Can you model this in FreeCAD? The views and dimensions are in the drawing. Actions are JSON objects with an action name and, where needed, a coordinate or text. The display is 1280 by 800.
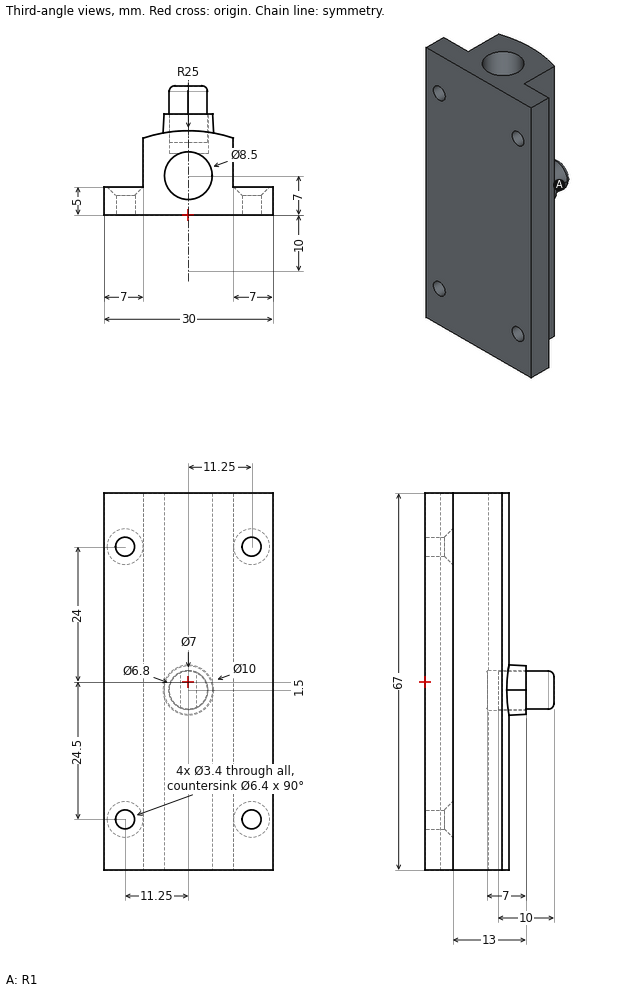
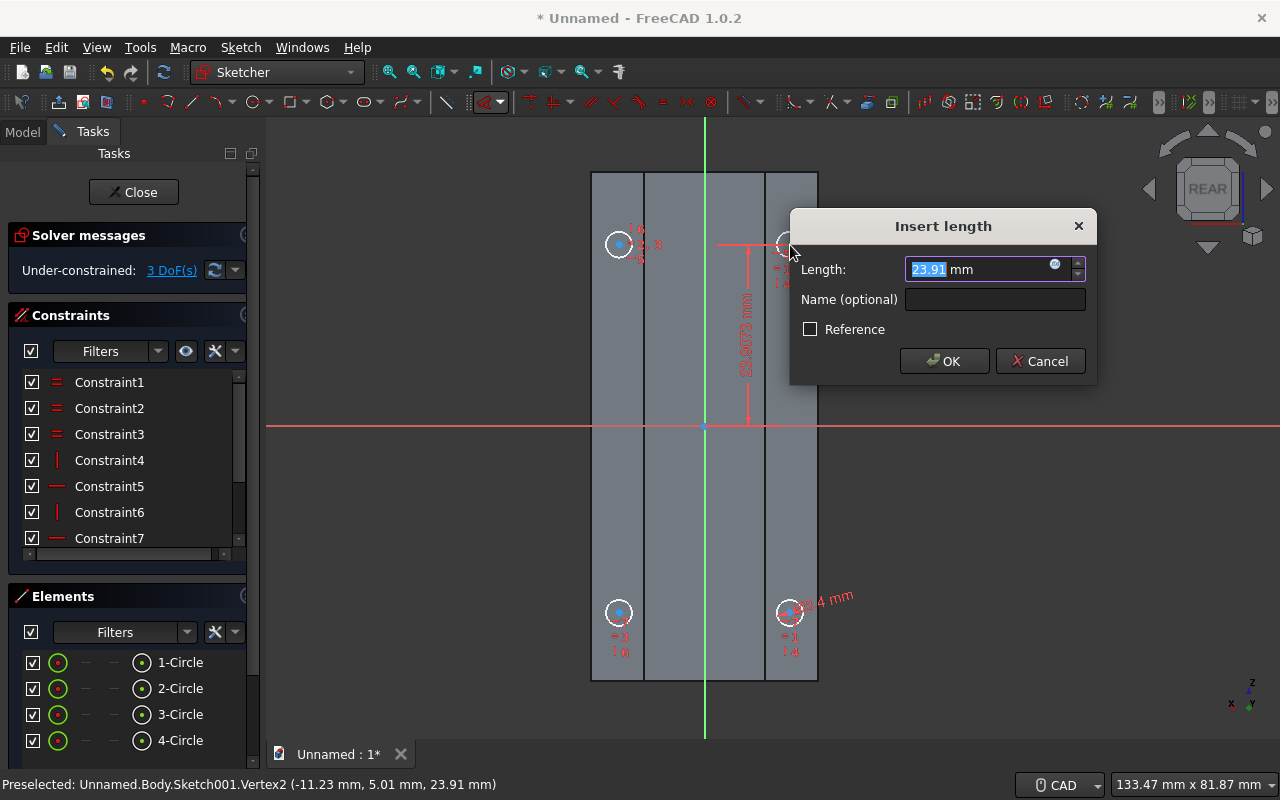
{"action": "type", "text": "24"}
{"action": "key", "text": "Return"}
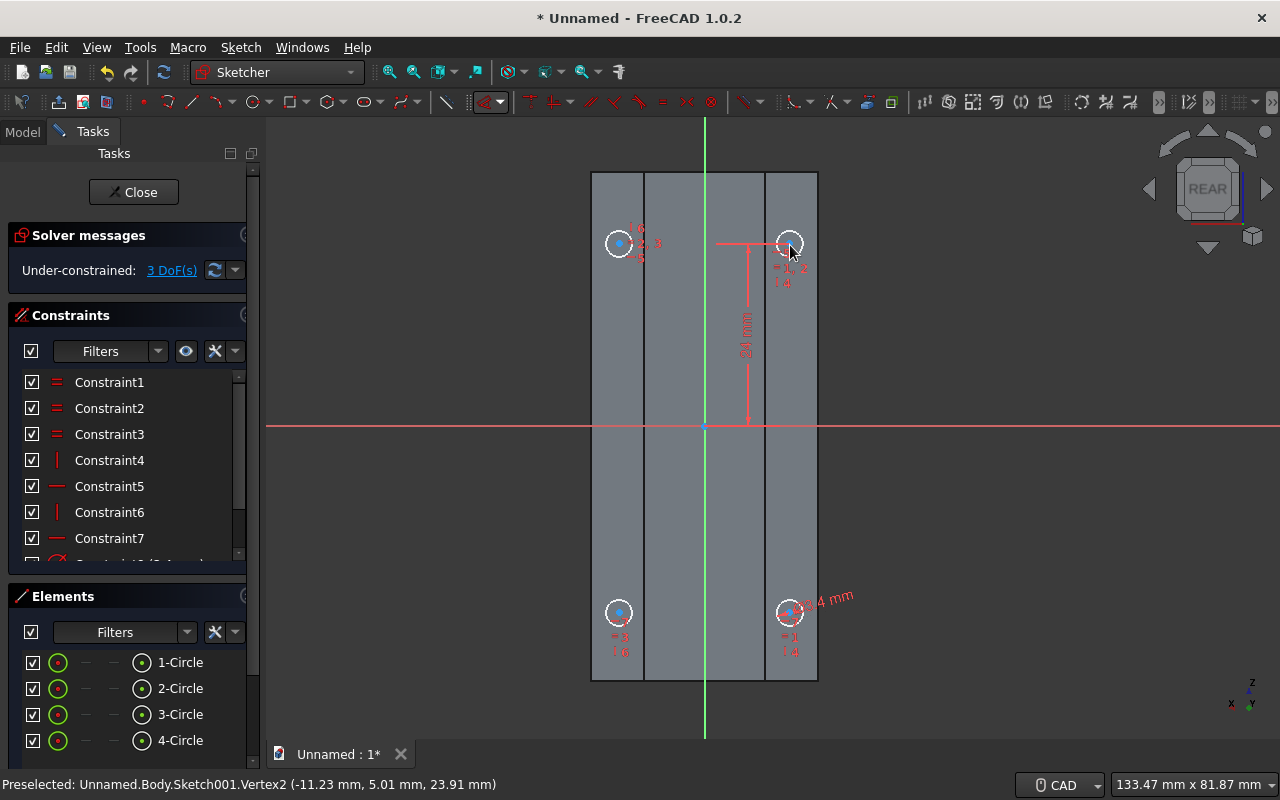
{"action": "left_click", "coordinate": [790, 613]}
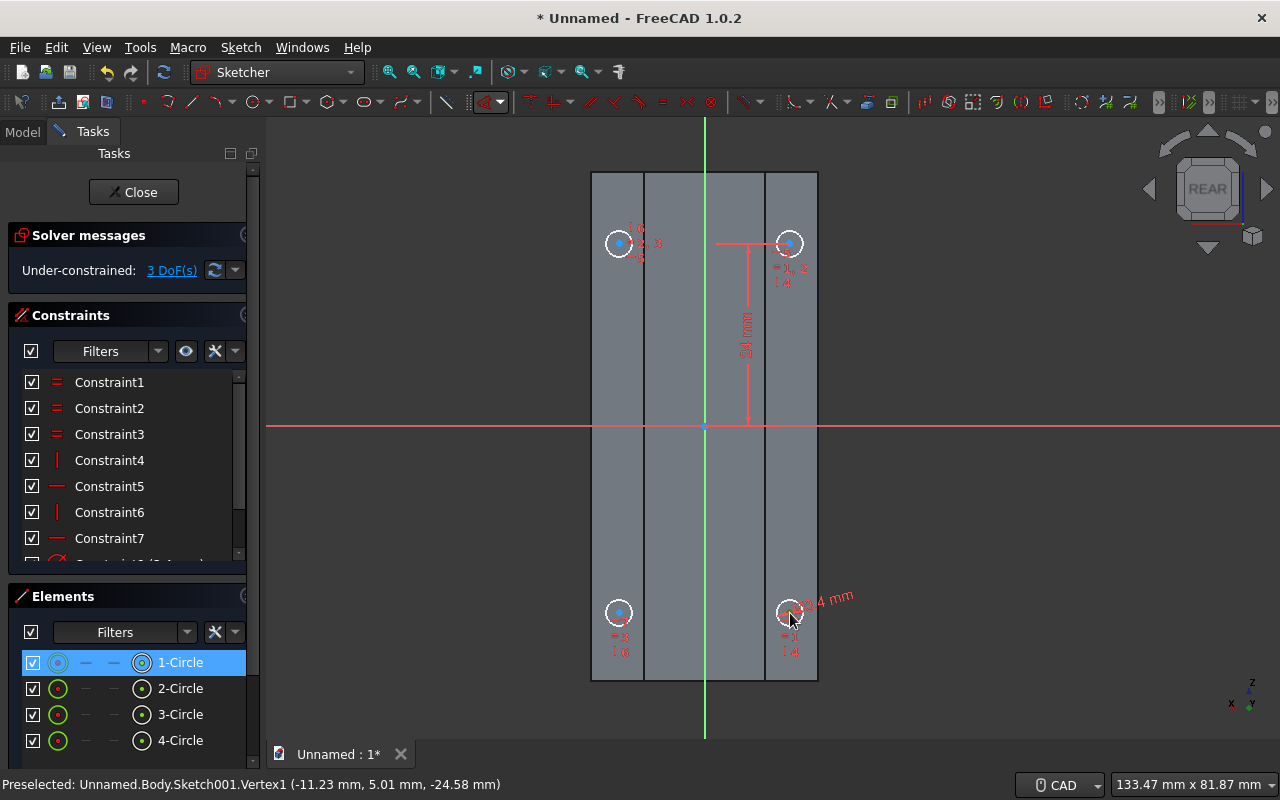
{"action": "key", "text": "i"}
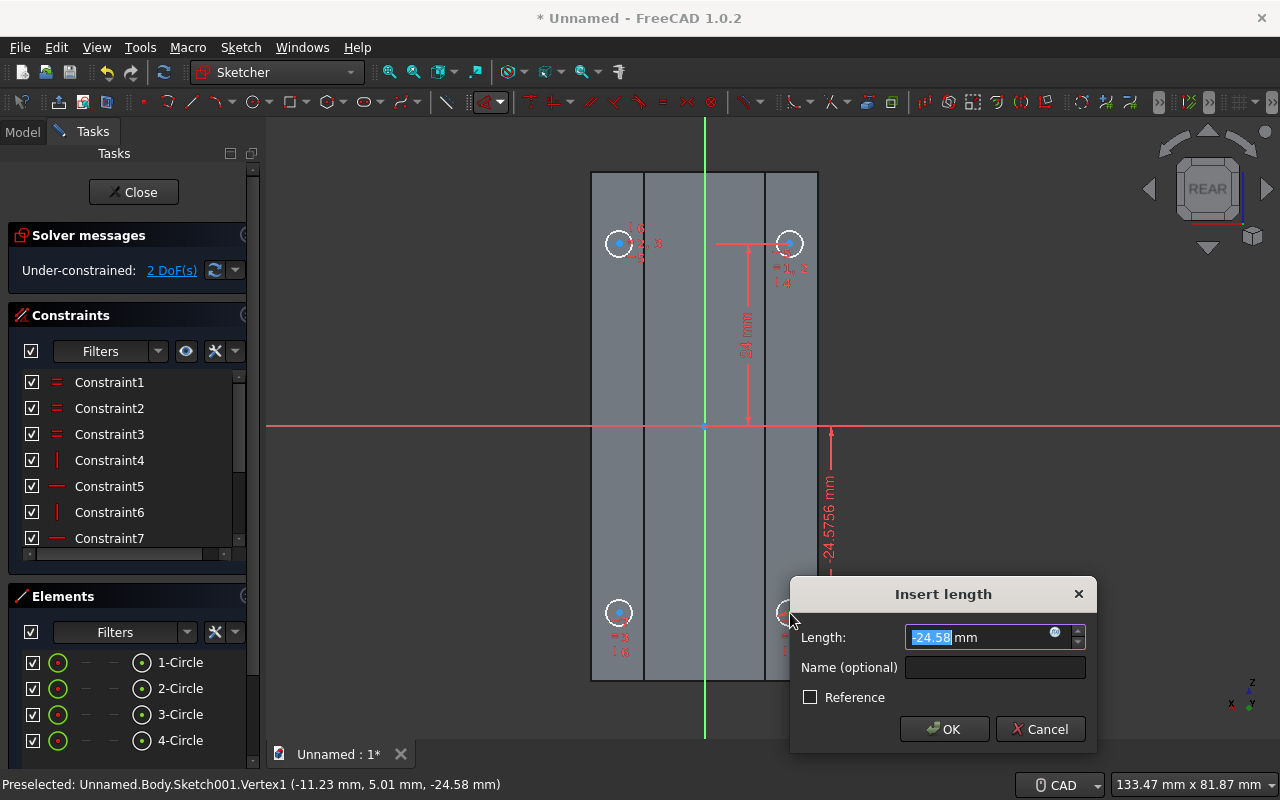
{"action": "type", "text": "-24.5"}
{"action": "key", "text": "Return"}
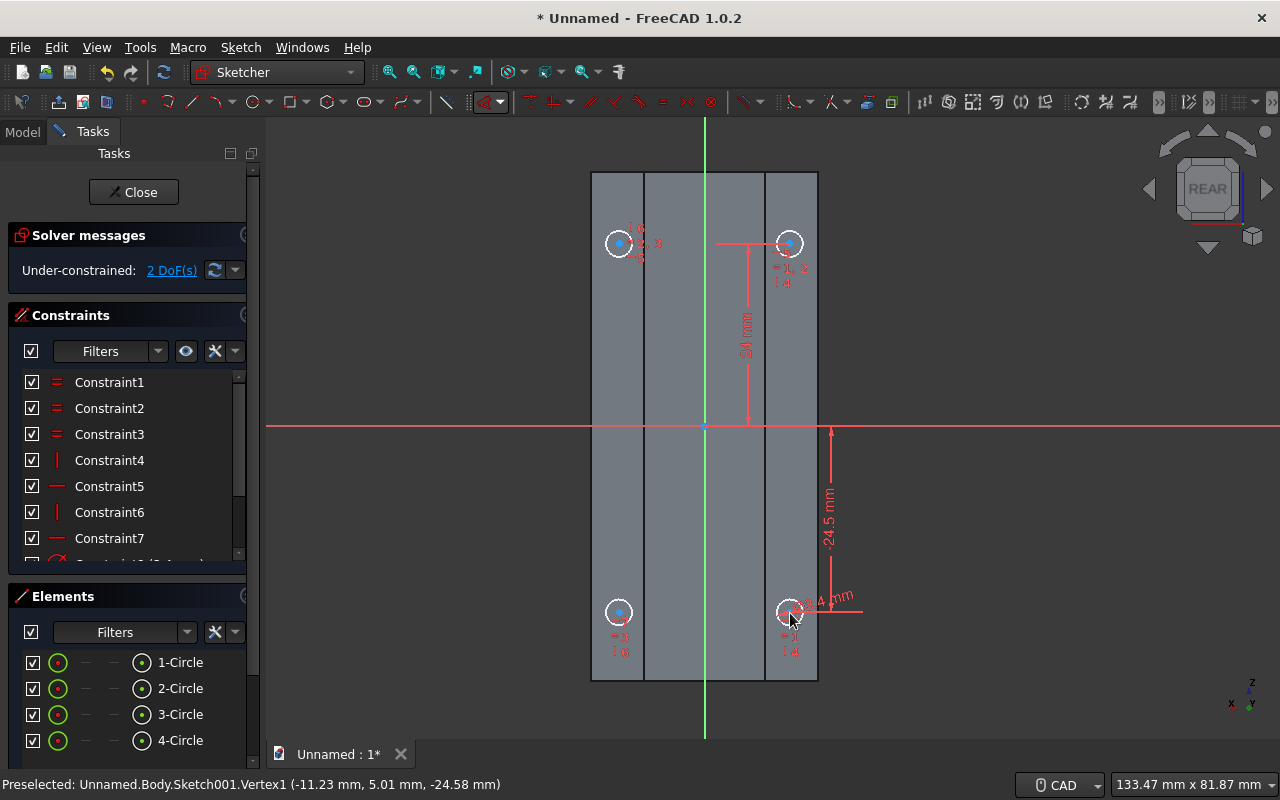
{"action": "left_click", "coordinate": [790, 612]}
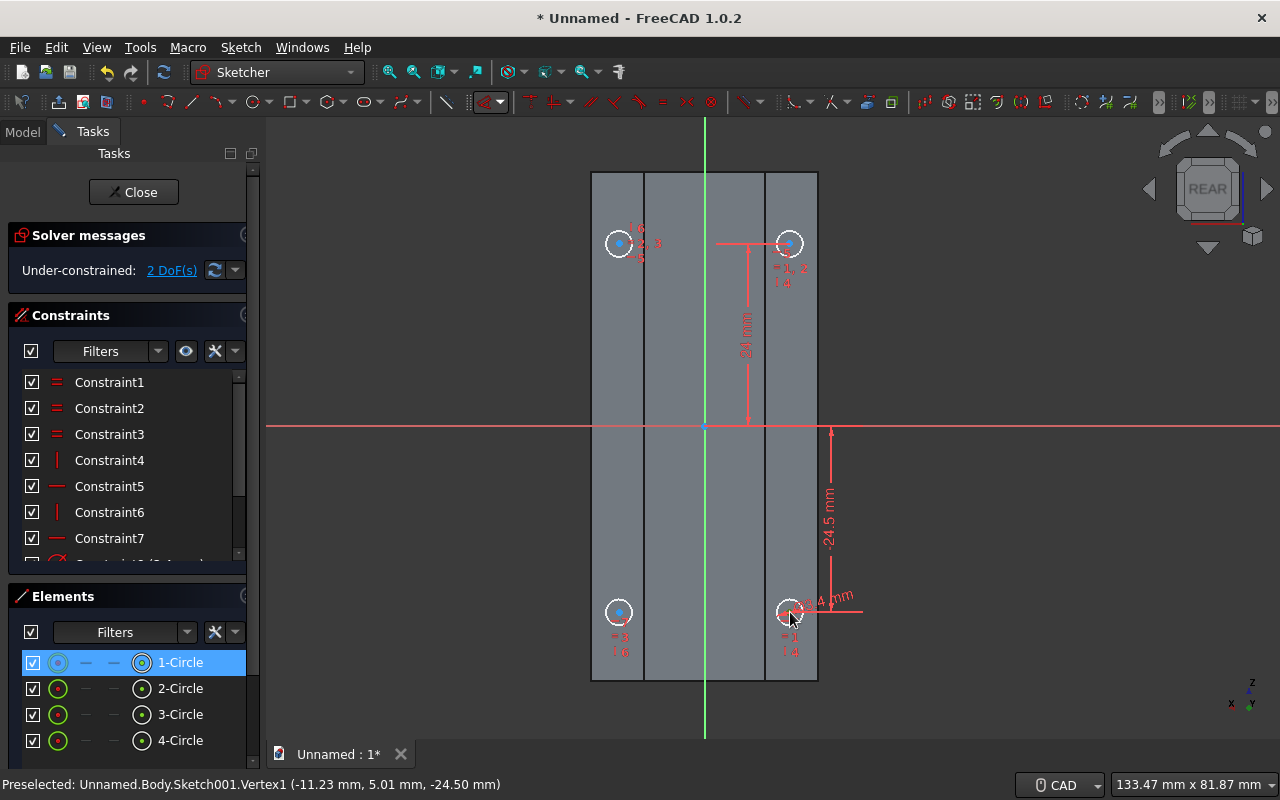
{"action": "key", "text": "l"}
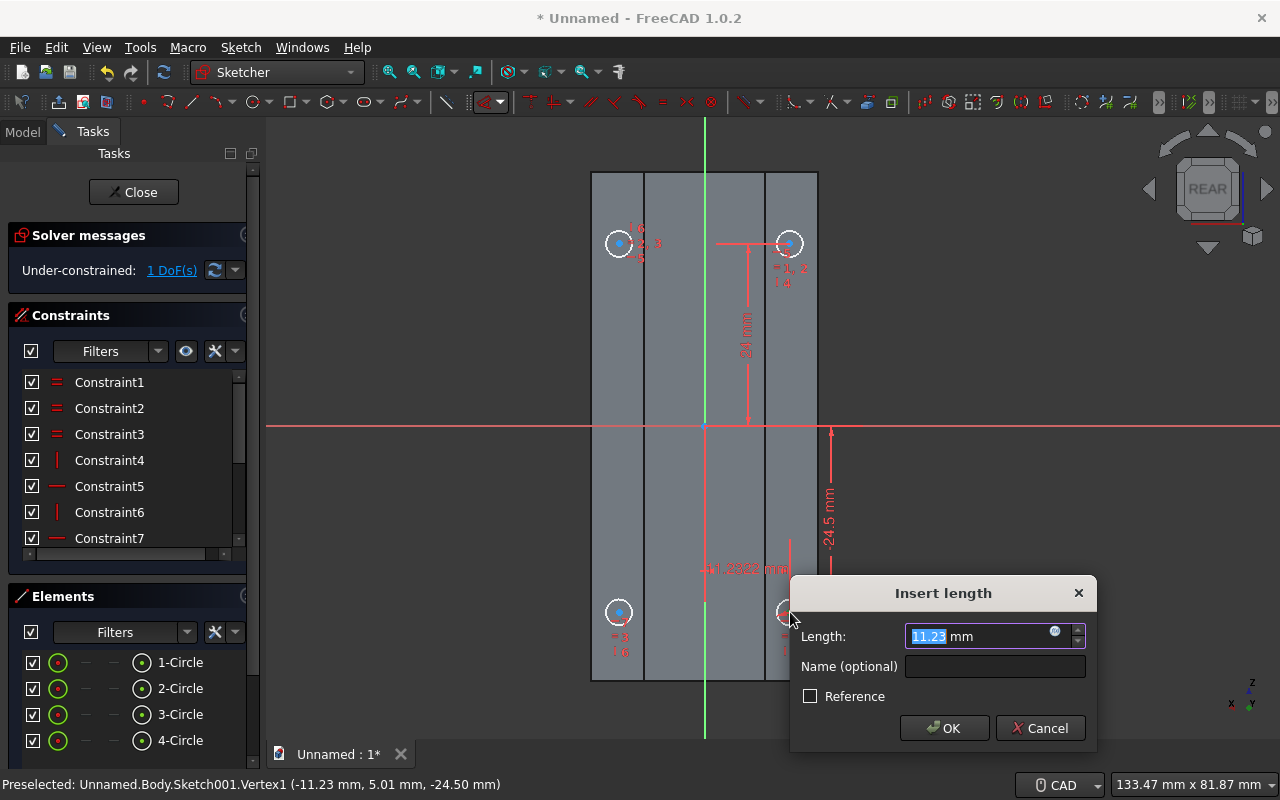
{"action": "type", "text": "11.25"}
{"action": "key", "text": "Return"}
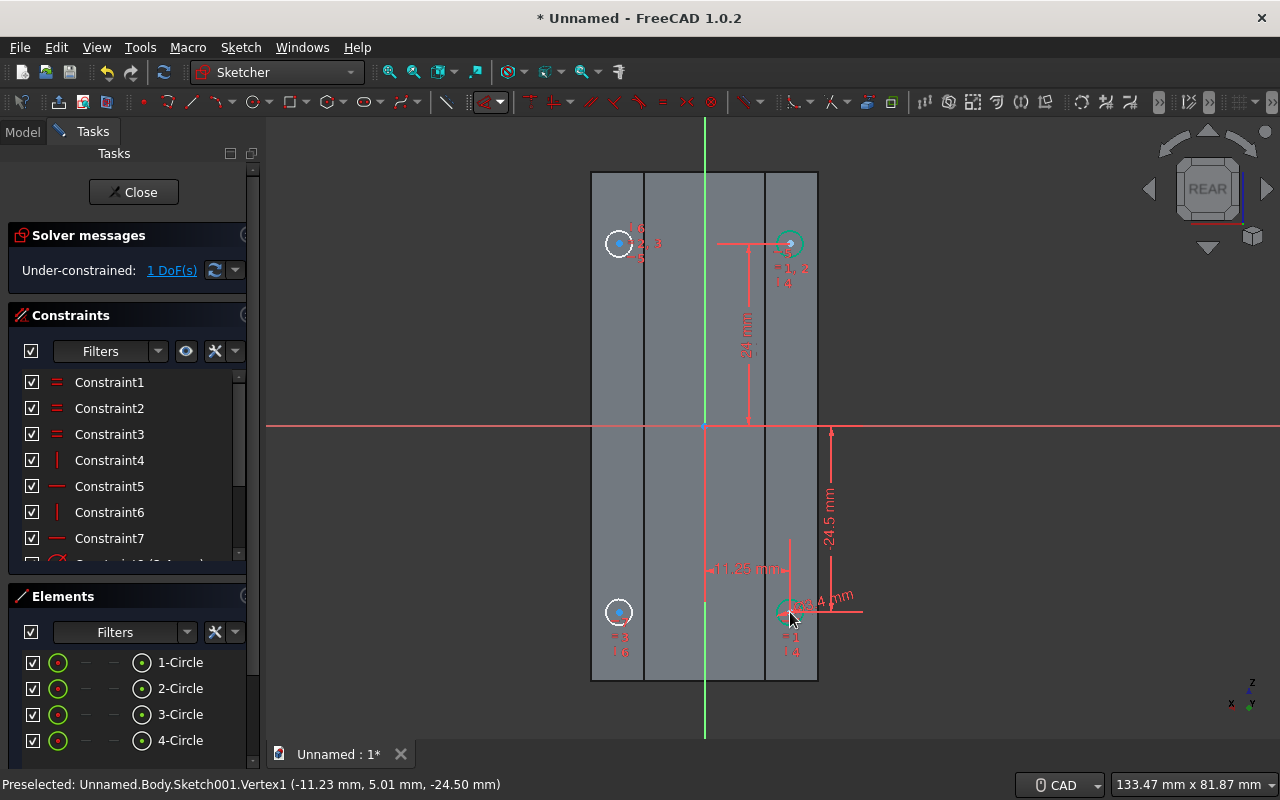
{"action": "left_click", "coordinate": [619, 244]}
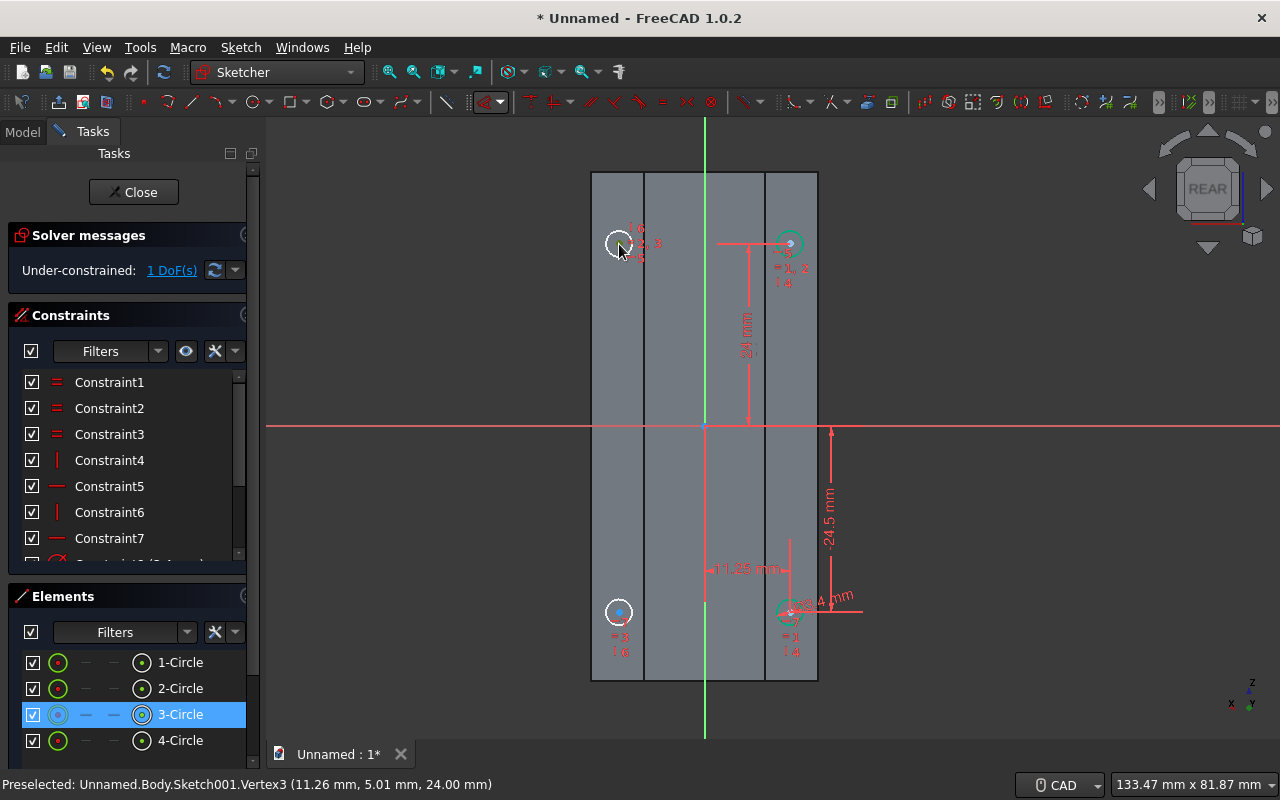
{"action": "key", "text": "l"}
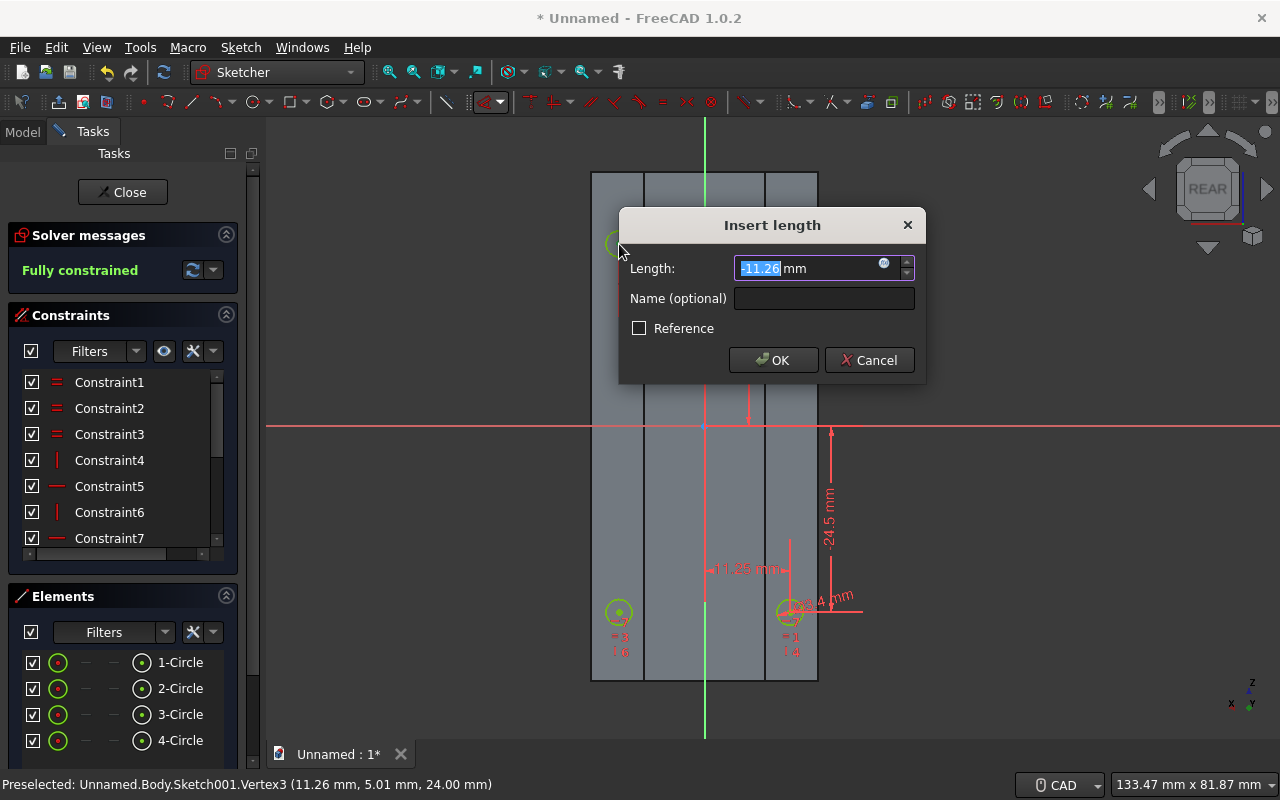
{"action": "type", "text": "-11.25"}
{"action": "key", "text": "Return"}